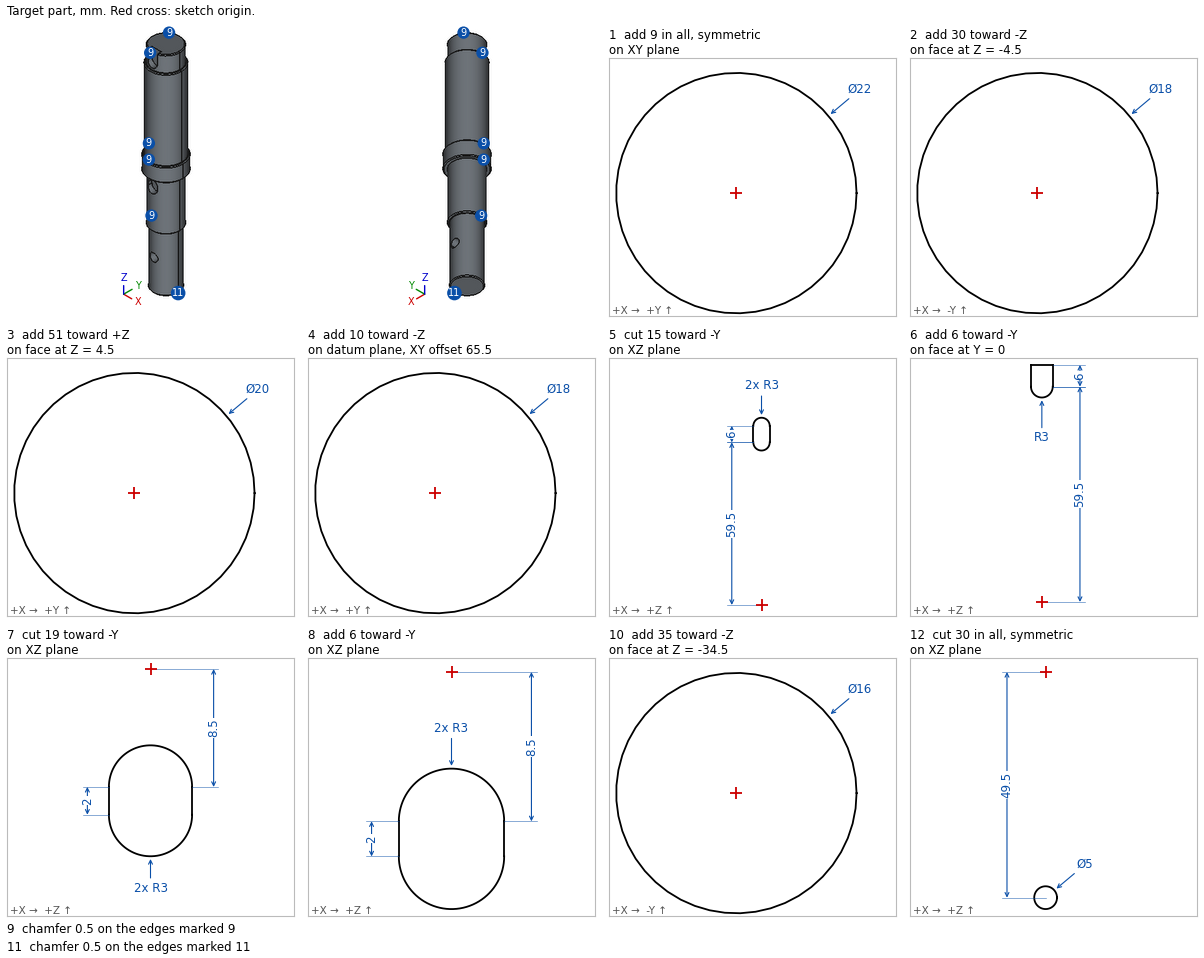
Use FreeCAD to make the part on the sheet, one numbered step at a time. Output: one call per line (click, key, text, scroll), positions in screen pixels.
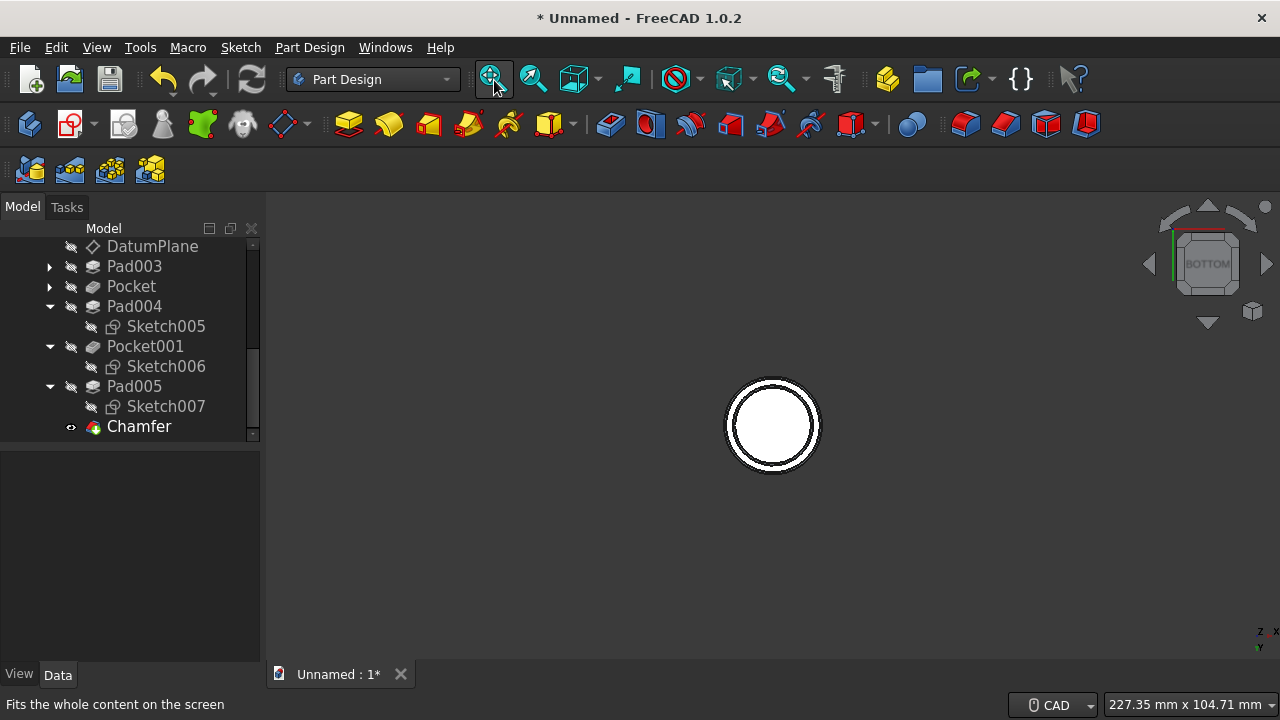
click(773, 424)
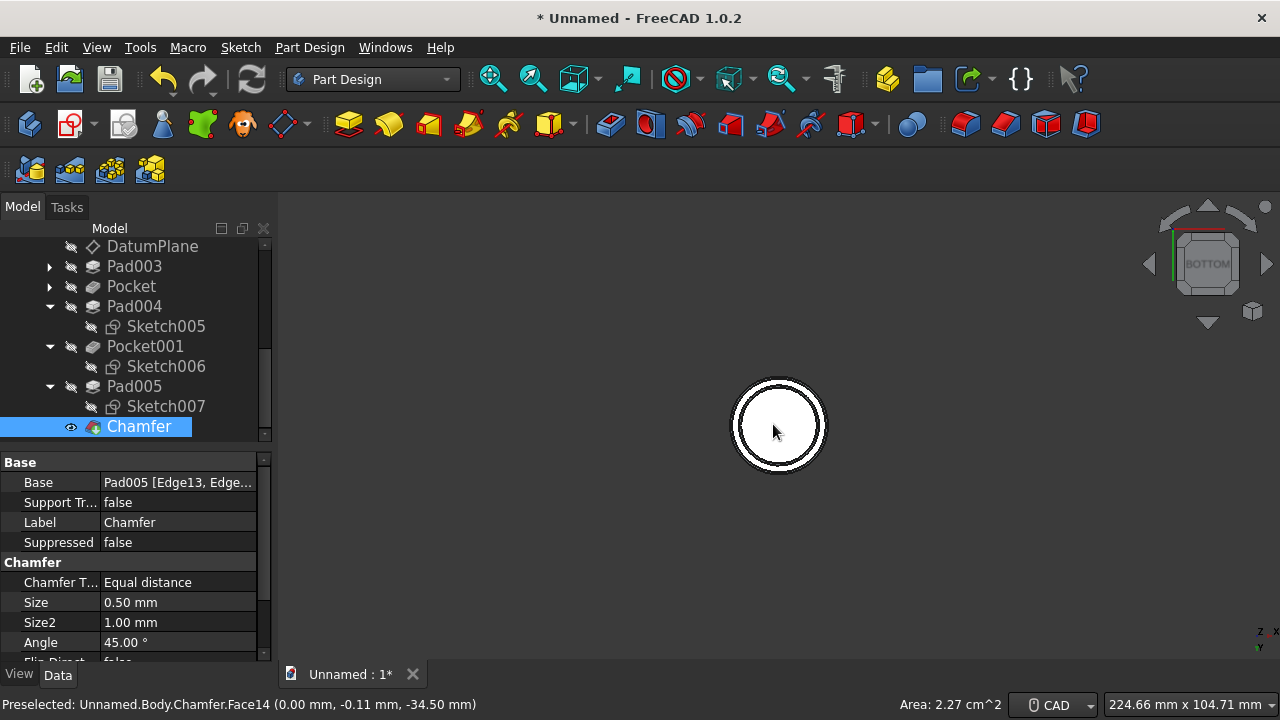
click(70, 124)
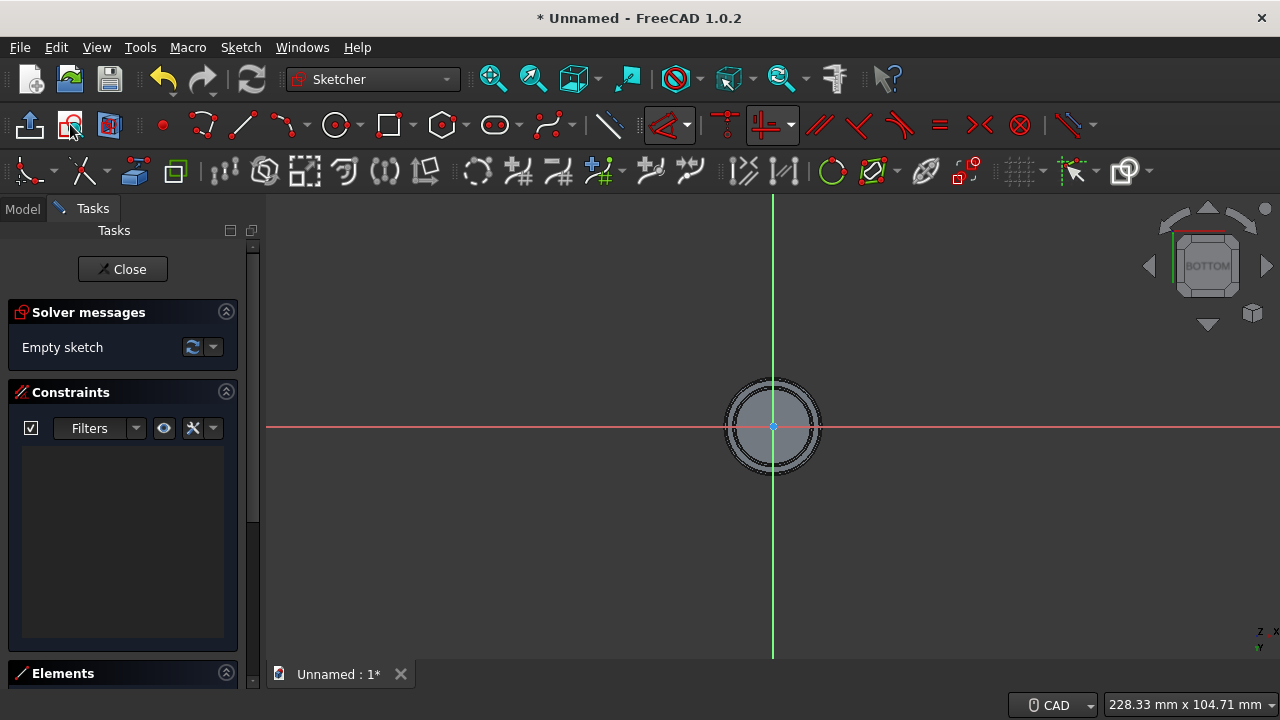
scroll(795, 426, up, 7)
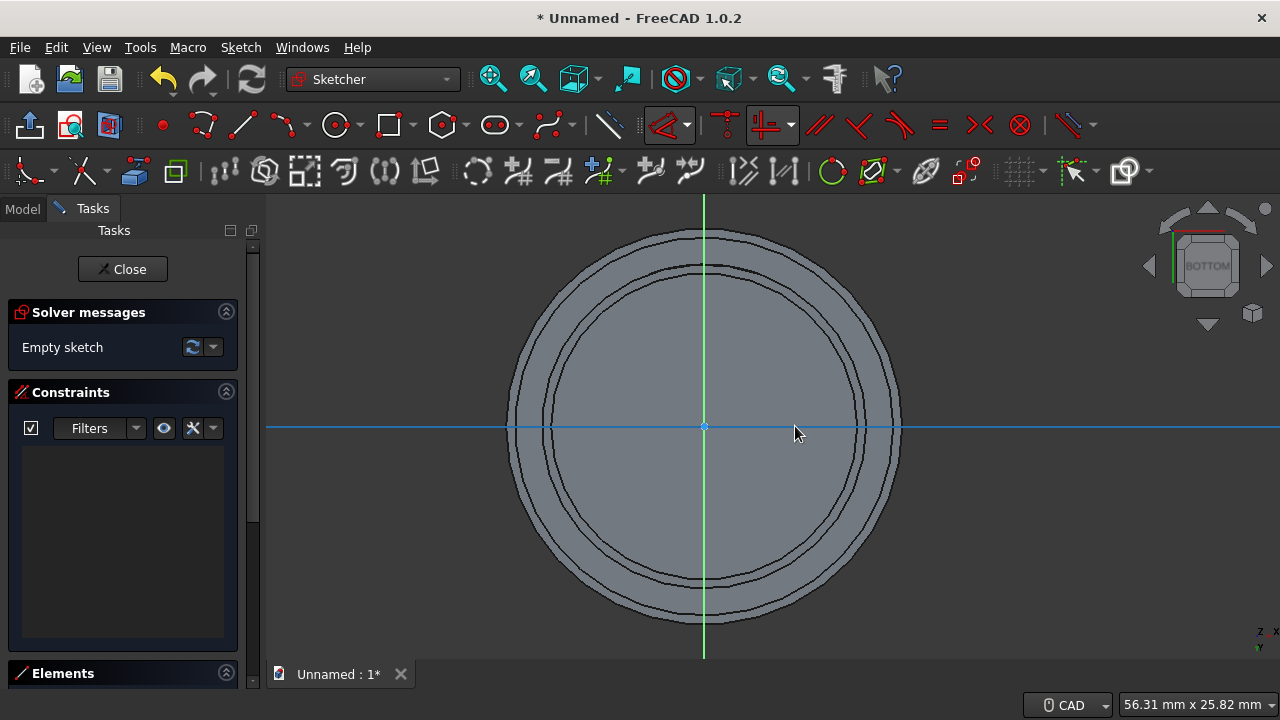
click(336, 126)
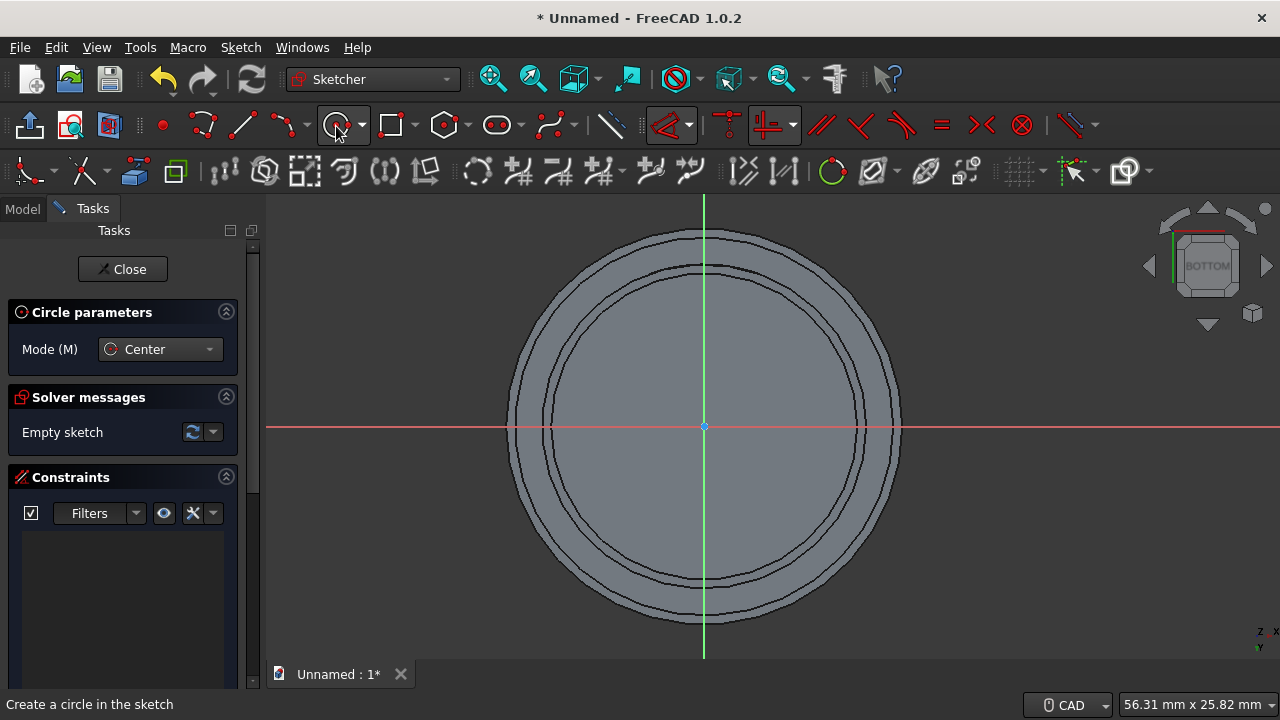
click(704, 426)
click(806, 325)
key(Escape)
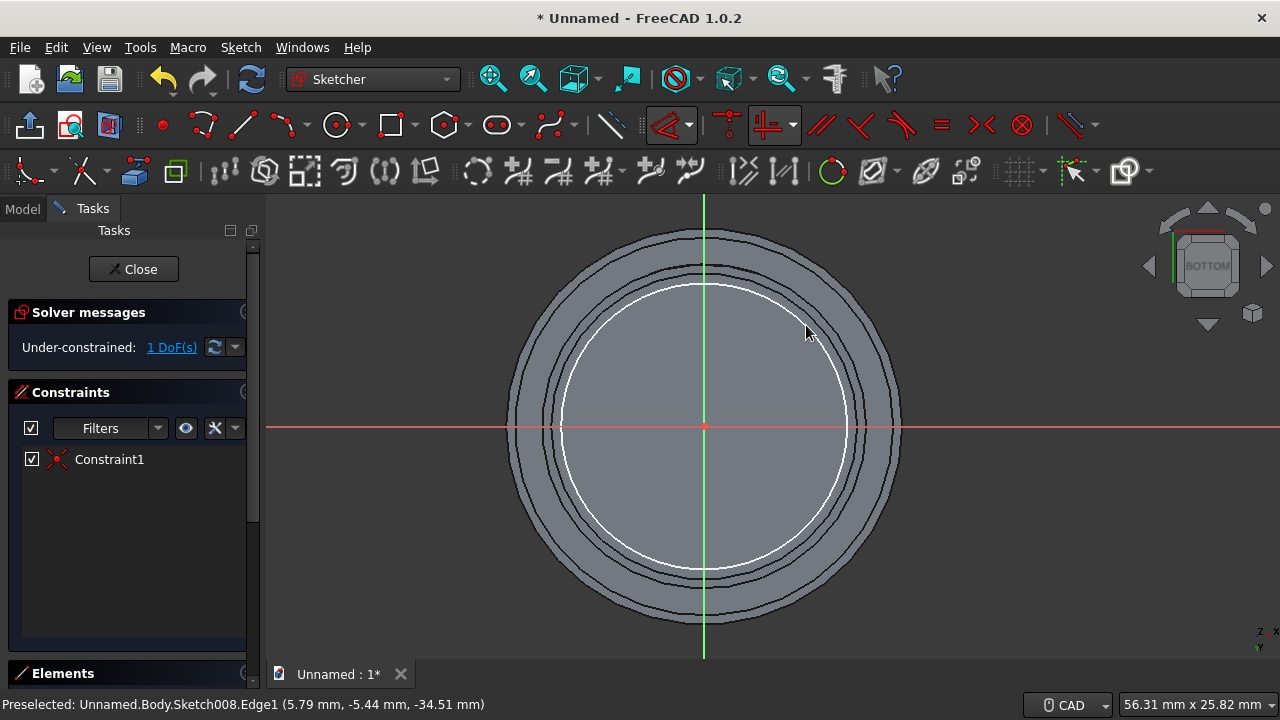
click(805, 325)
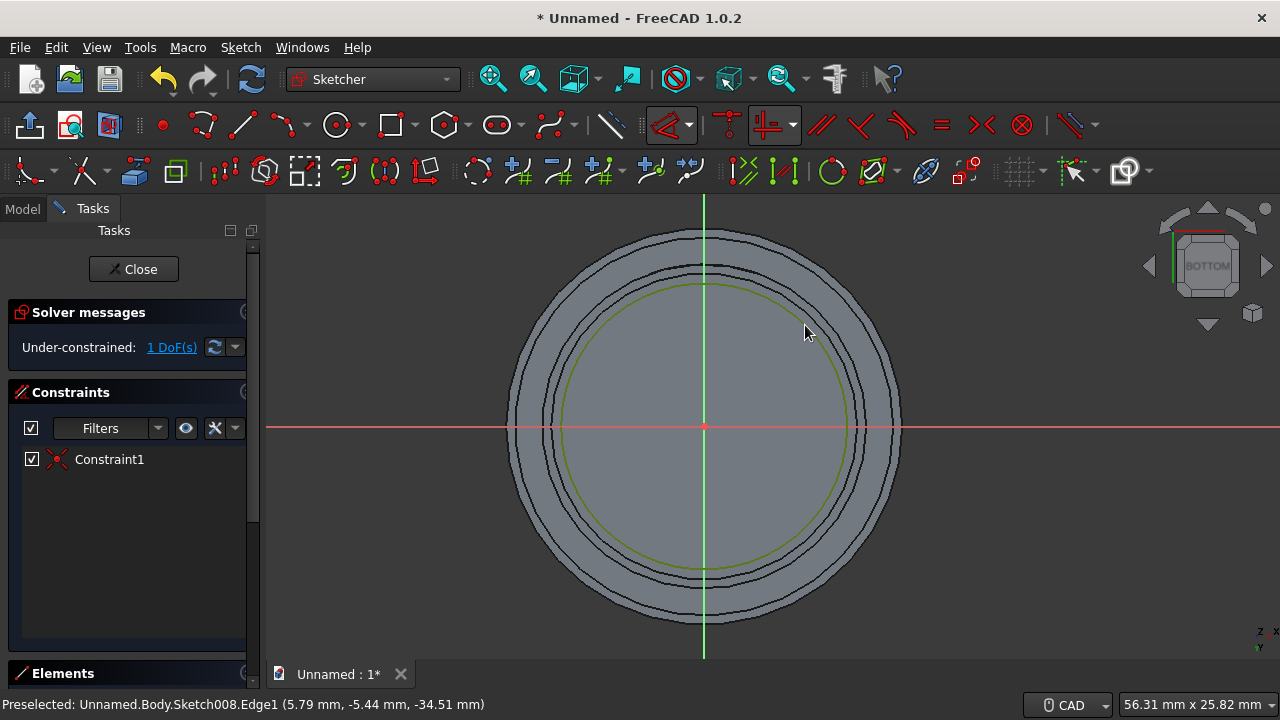
click(692, 126)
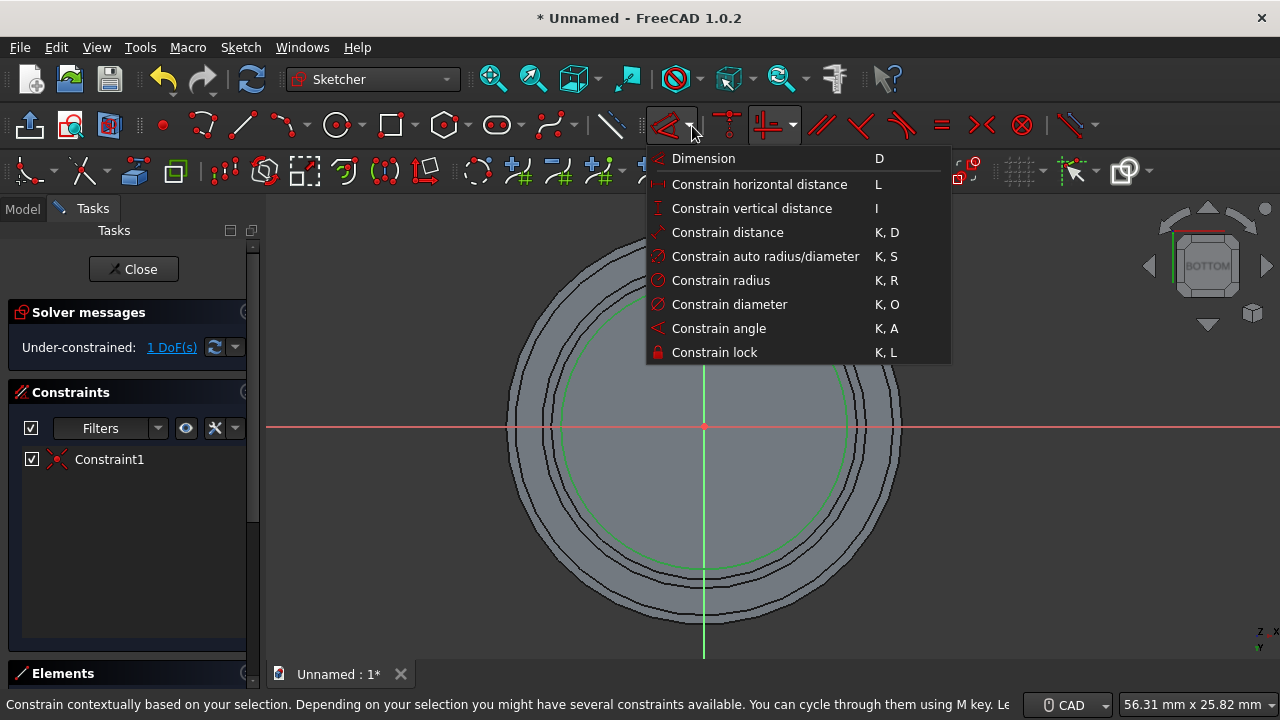
click(799, 304)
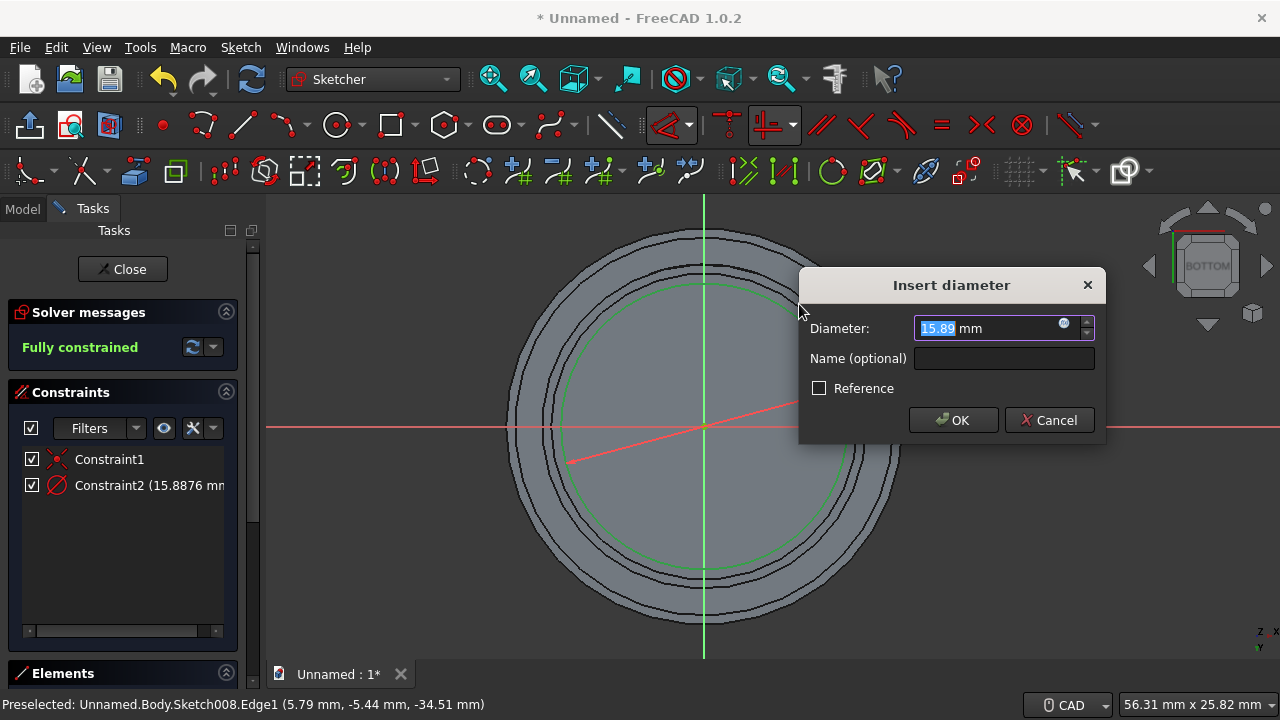
text(16)
key(Return)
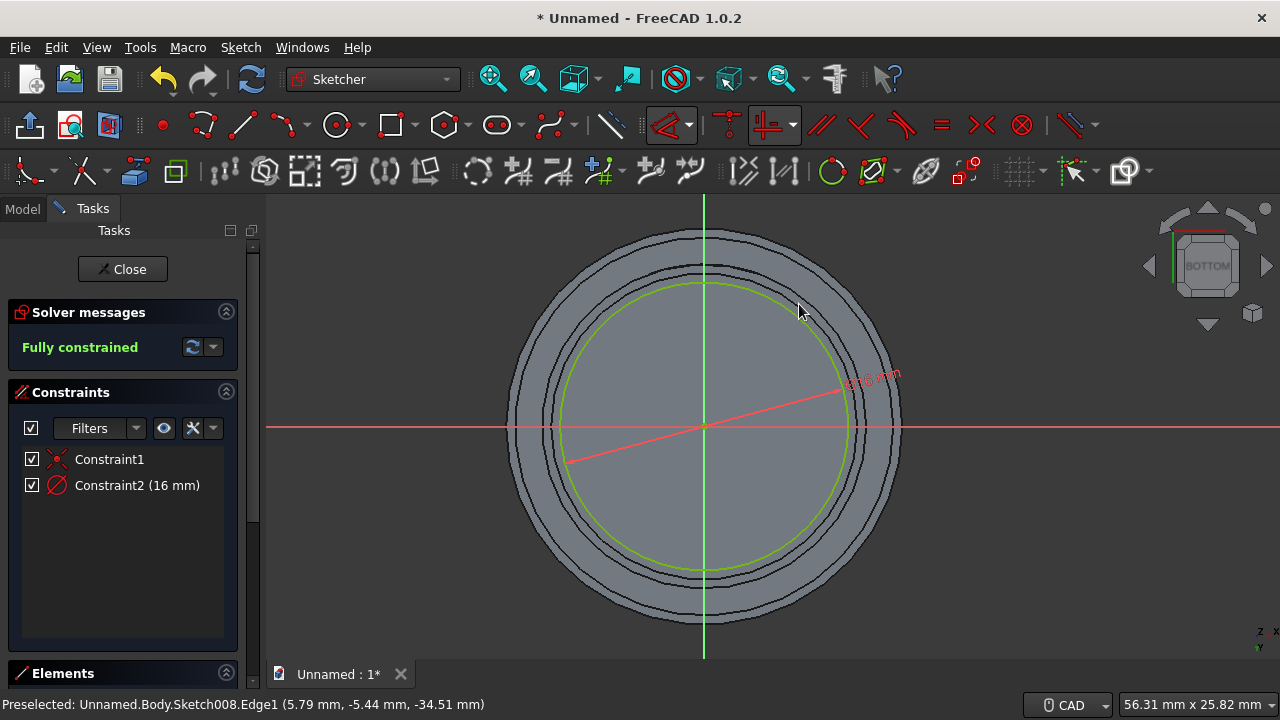
click(123, 269)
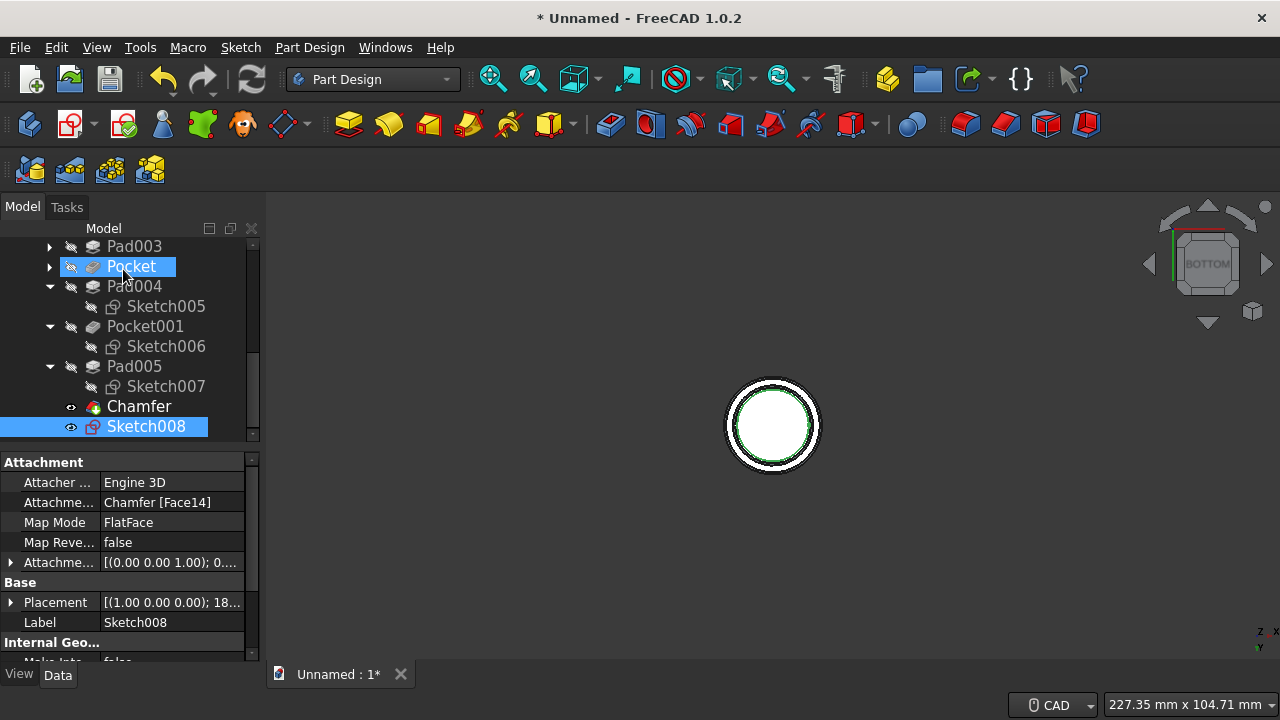
click(350, 124)